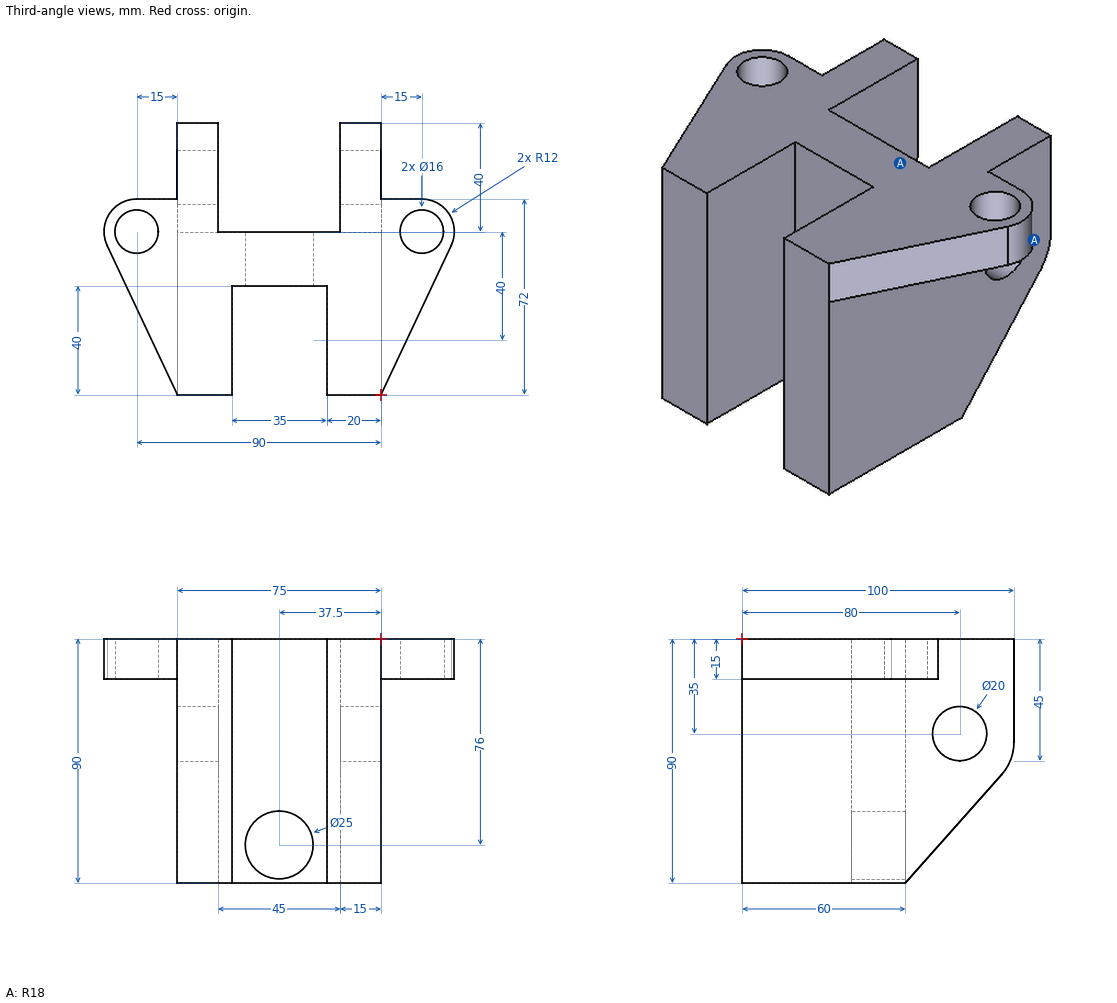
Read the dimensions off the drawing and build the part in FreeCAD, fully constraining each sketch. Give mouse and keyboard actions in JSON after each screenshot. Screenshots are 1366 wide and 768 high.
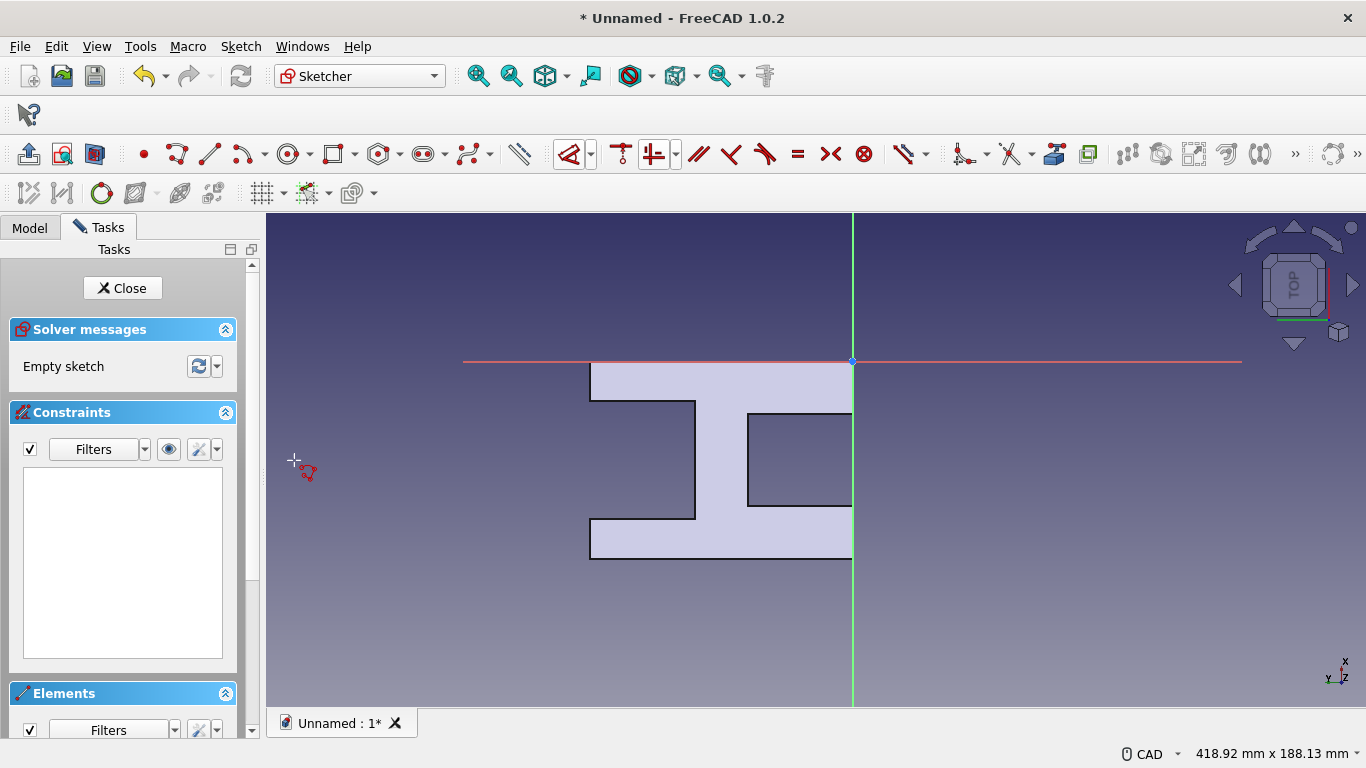
{"action": "left_click", "coordinate": [664, 322]}
{"action": "left_click", "coordinate": [664, 362]}
{"action": "left_click", "coordinate": [853, 362]}
{"action": "left_click", "coordinate": [709, 294]}
{"action": "right_click", "coordinate": [709, 294]}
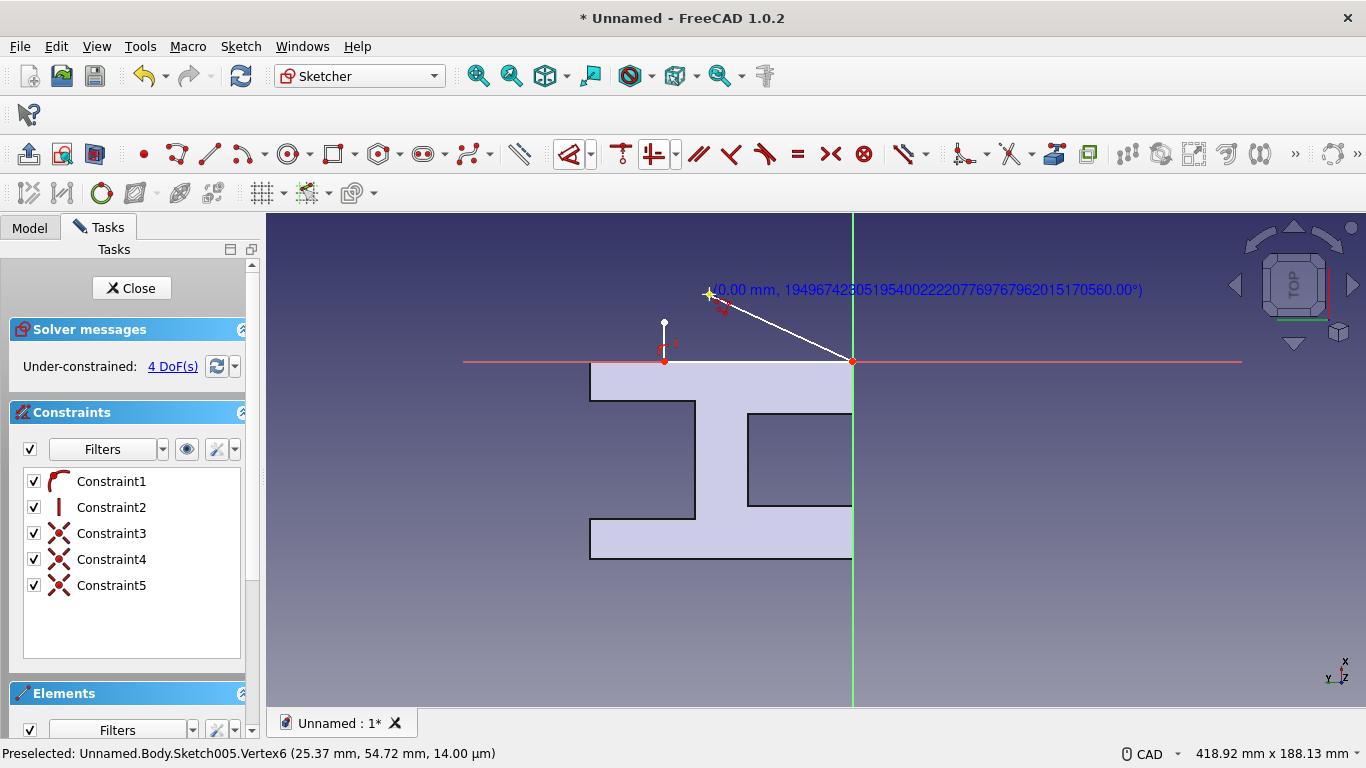
{"action": "left_click", "coordinate": [264, 154]}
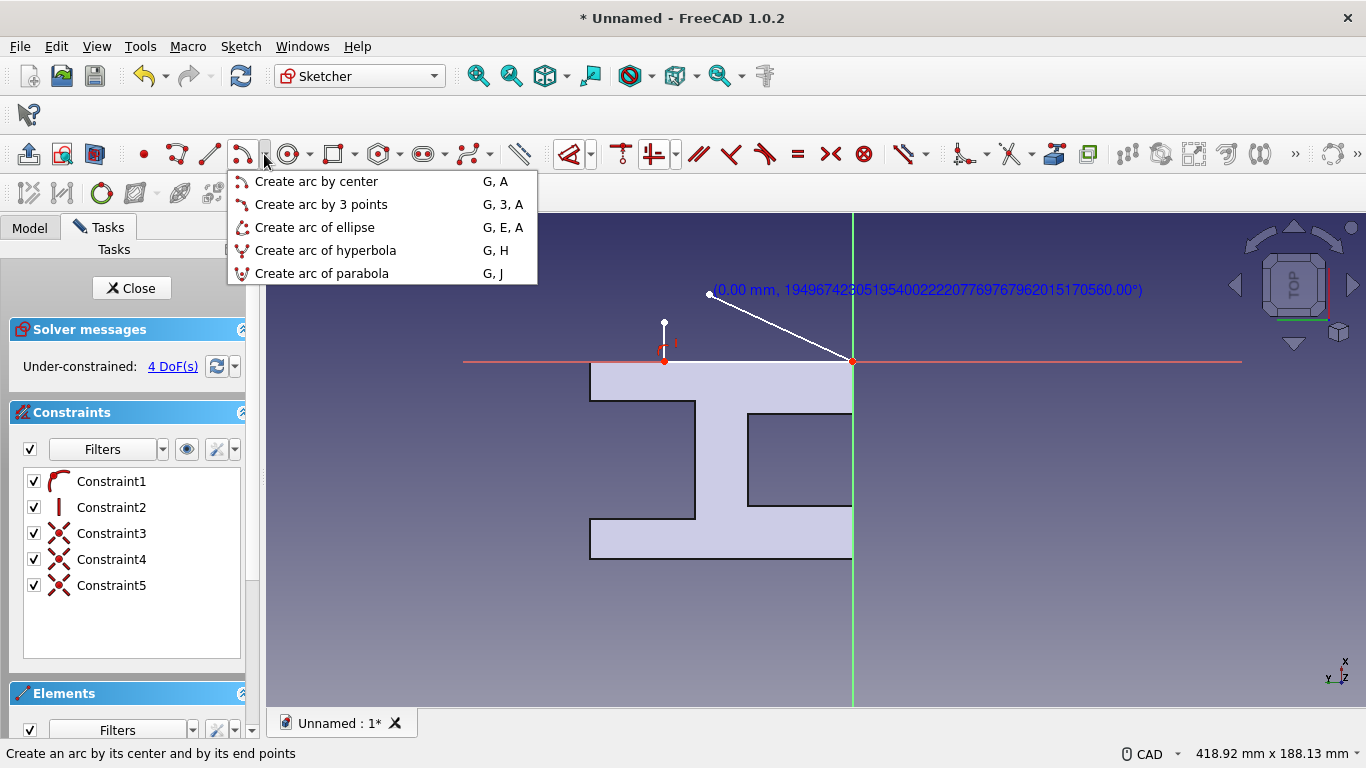
{"action": "left_click", "coordinate": [382, 204]}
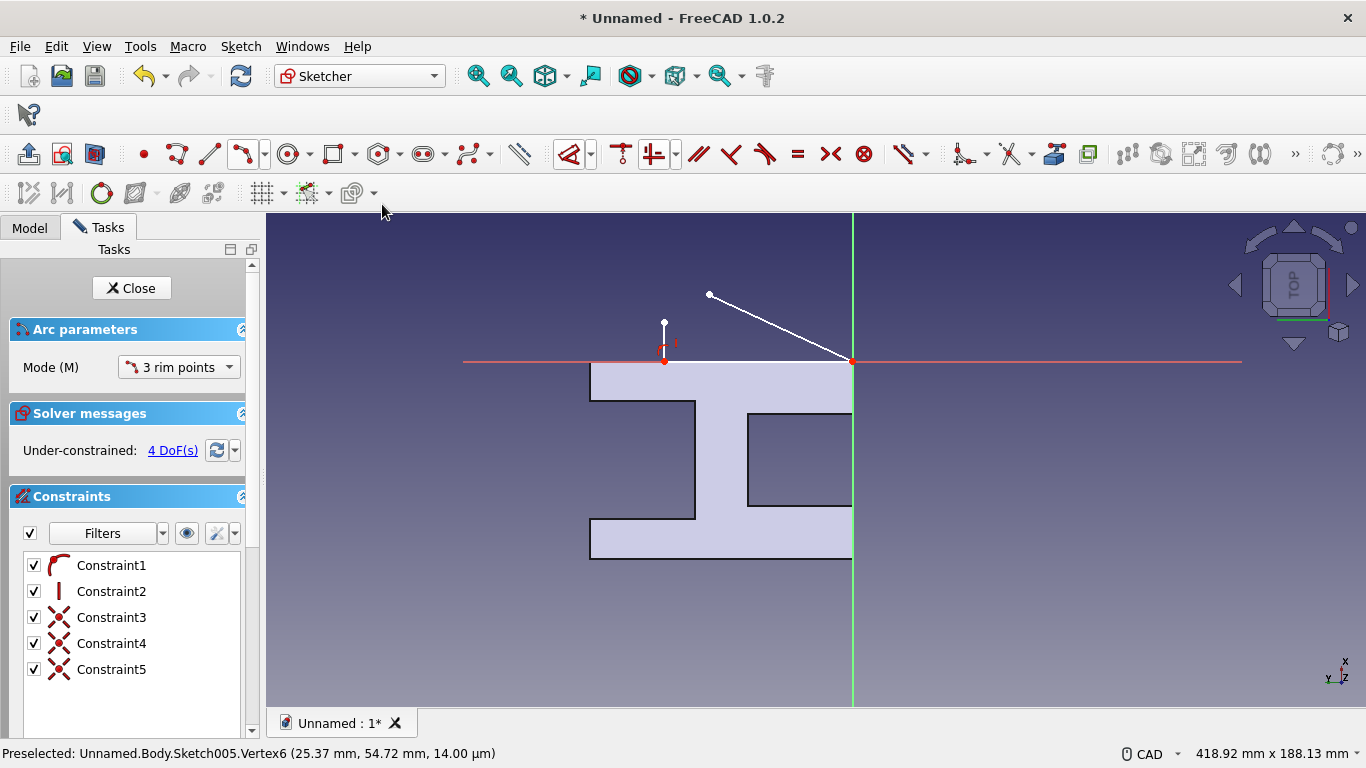
{"action": "left_click", "coordinate": [709, 295]}
{"action": "left_click", "coordinate": [664, 323]}
{"action": "left_click", "coordinate": [678, 296]}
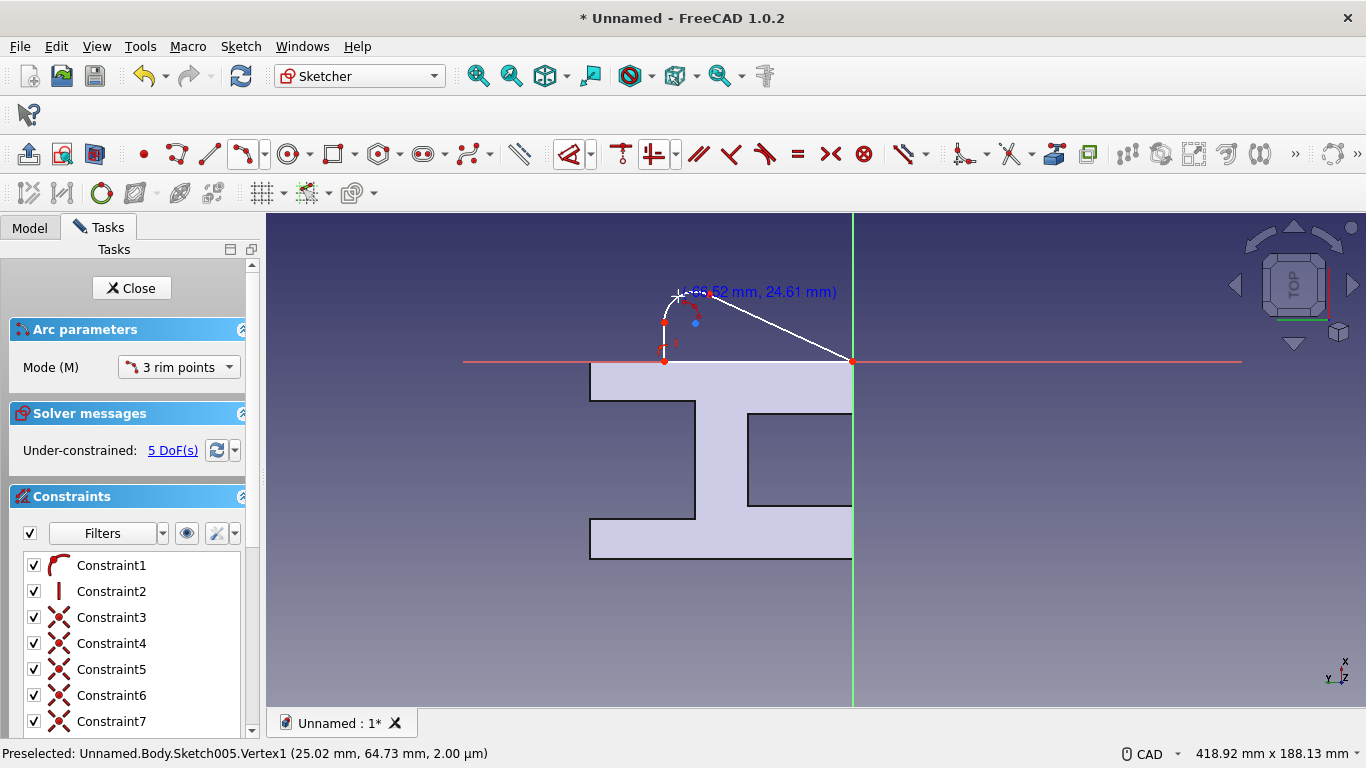
{"action": "left_click", "coordinate": [177, 154]}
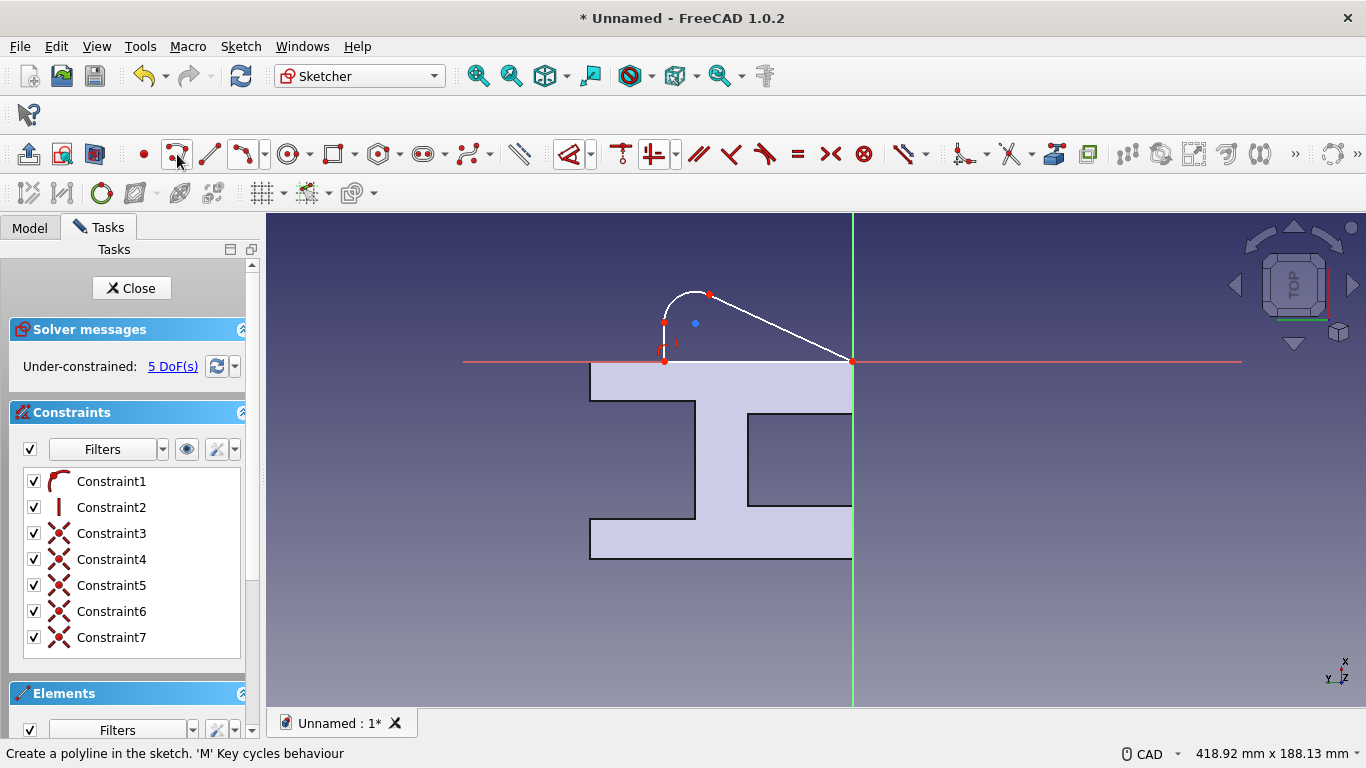
{"action": "left_click", "coordinate": [709, 626]}
{"action": "left_click", "coordinate": [853, 559]}
{"action": "left_click", "coordinate": [664, 559]}
{"action": "left_click", "coordinate": [664, 598]}
{"action": "right_click", "coordinate": [664, 598]}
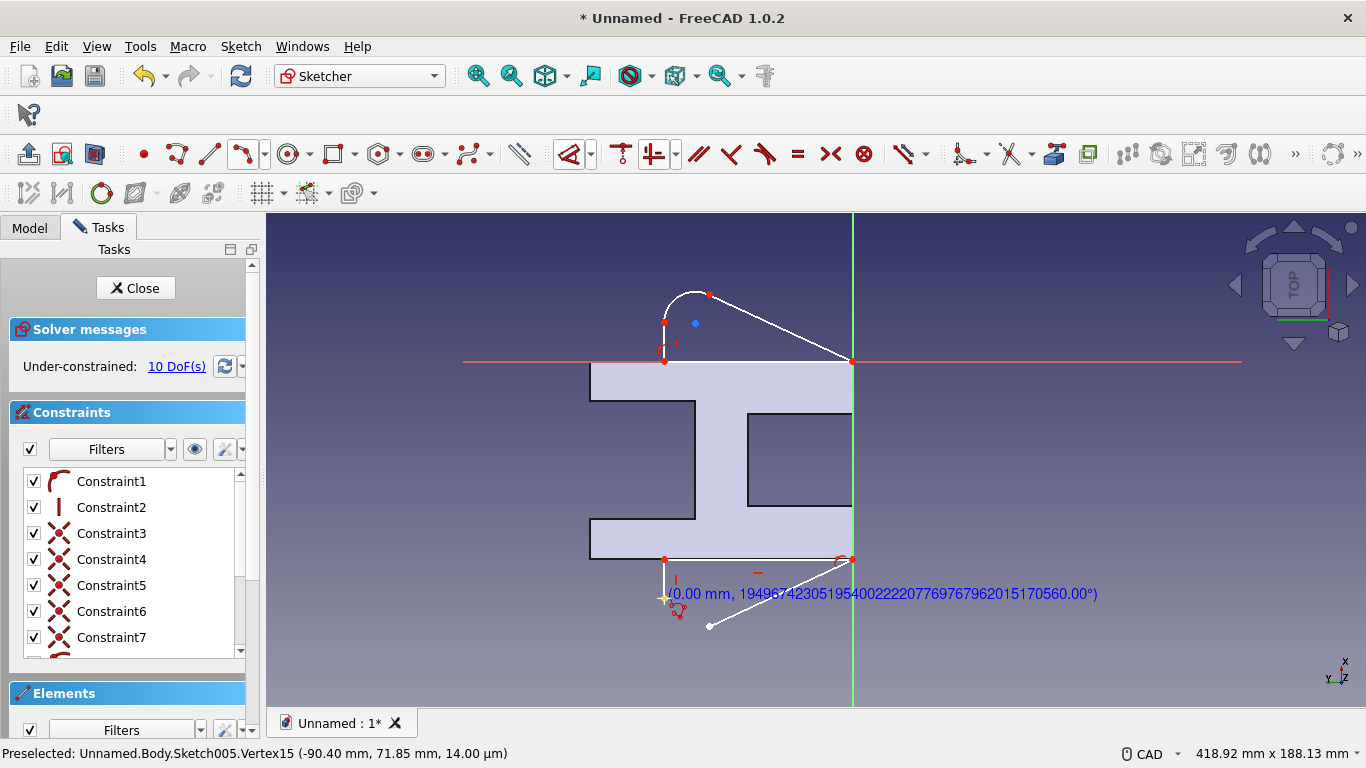
{"action": "left_click", "coordinate": [242, 154]}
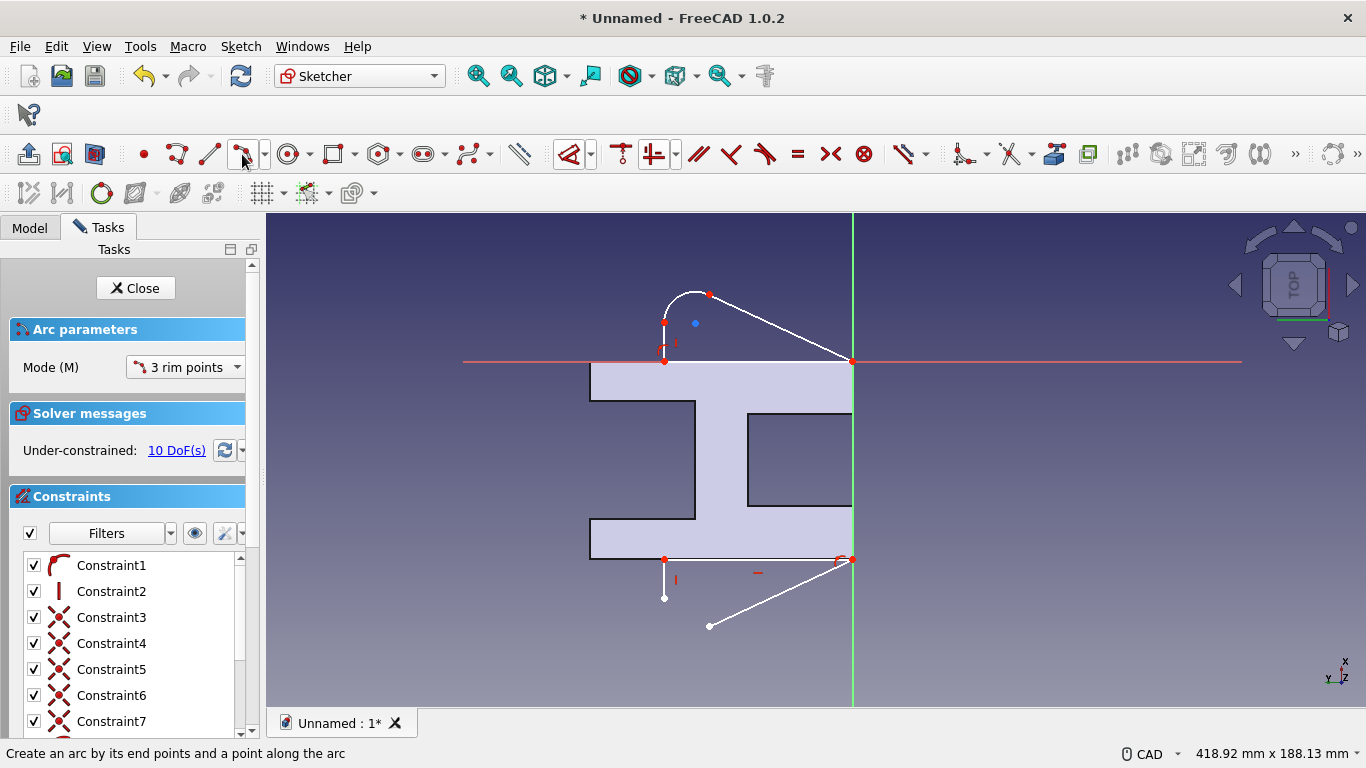
{"action": "left_click", "coordinate": [664, 599]}
{"action": "left_click", "coordinate": [709, 627]}
{"action": "left_click", "coordinate": [678, 625]}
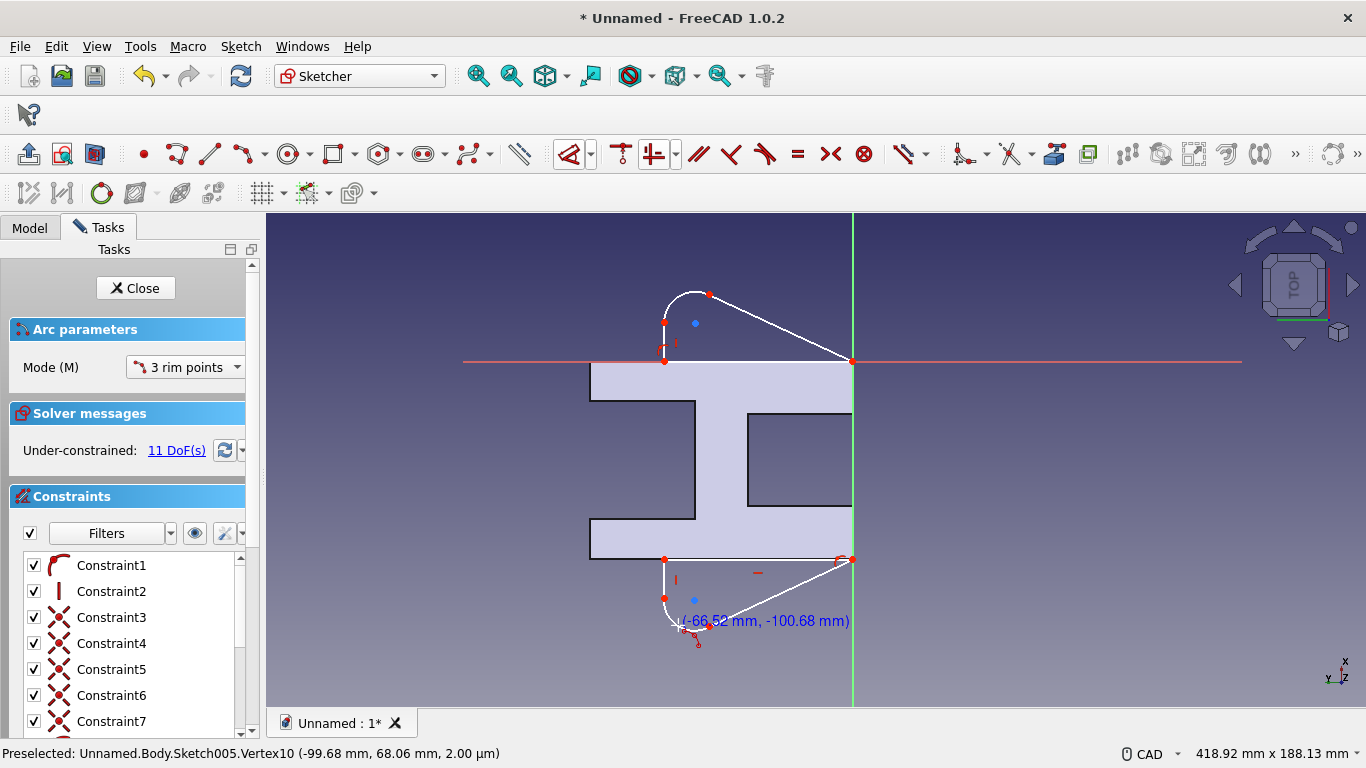
{"action": "key", "text": "g c"}